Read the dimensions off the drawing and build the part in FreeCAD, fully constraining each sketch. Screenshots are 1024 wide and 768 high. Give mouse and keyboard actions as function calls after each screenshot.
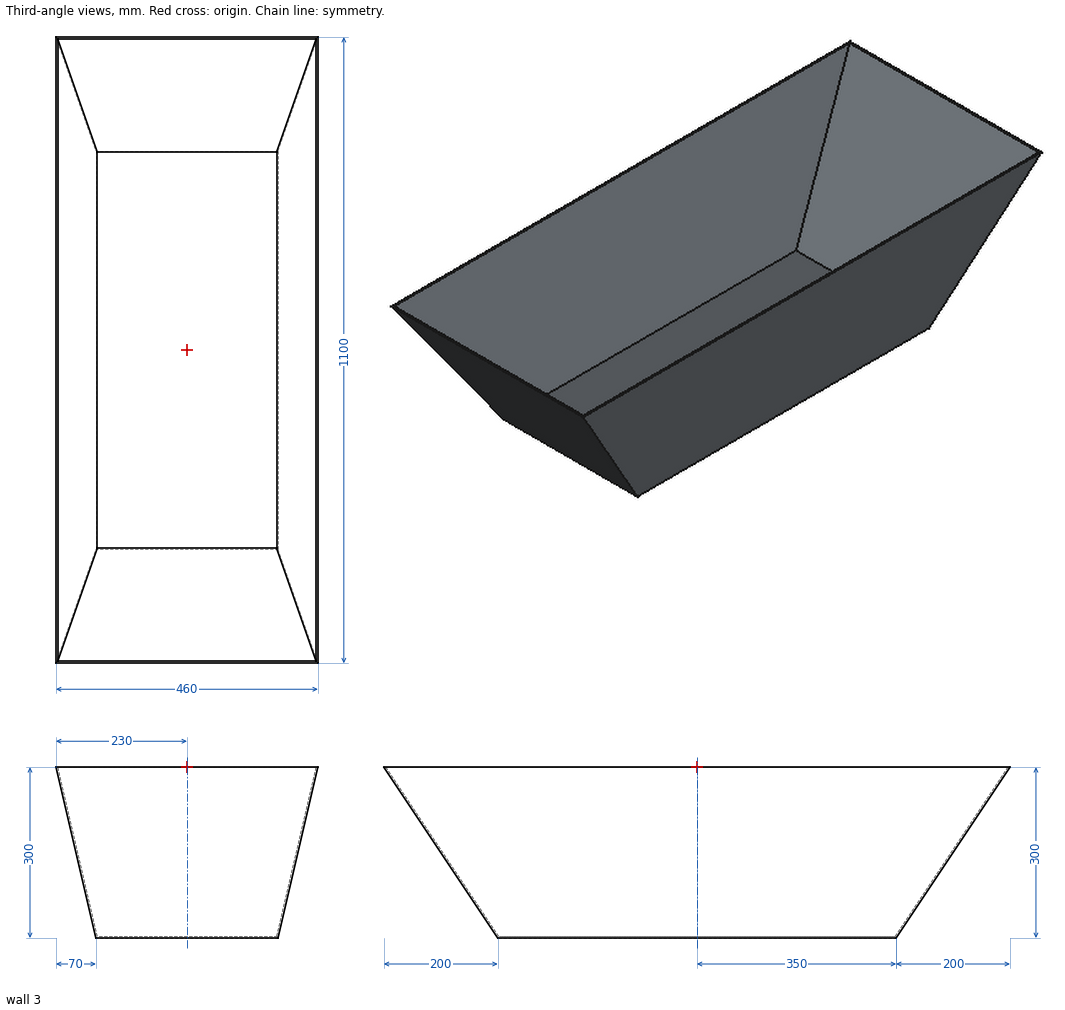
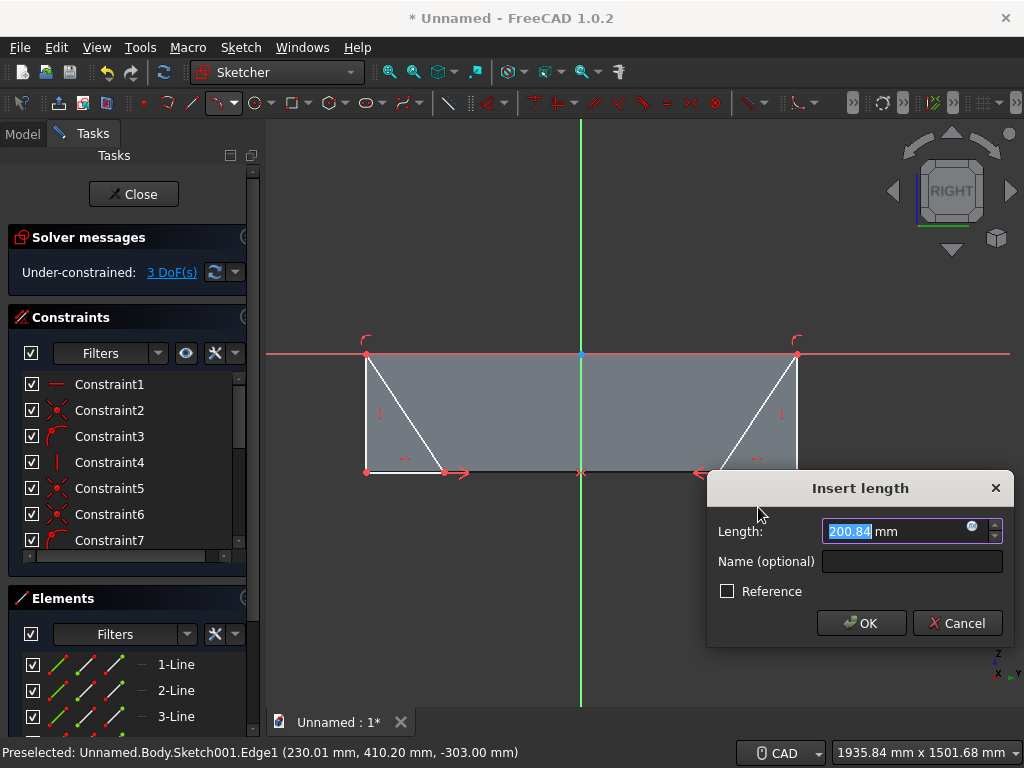
text(200)
key(Return)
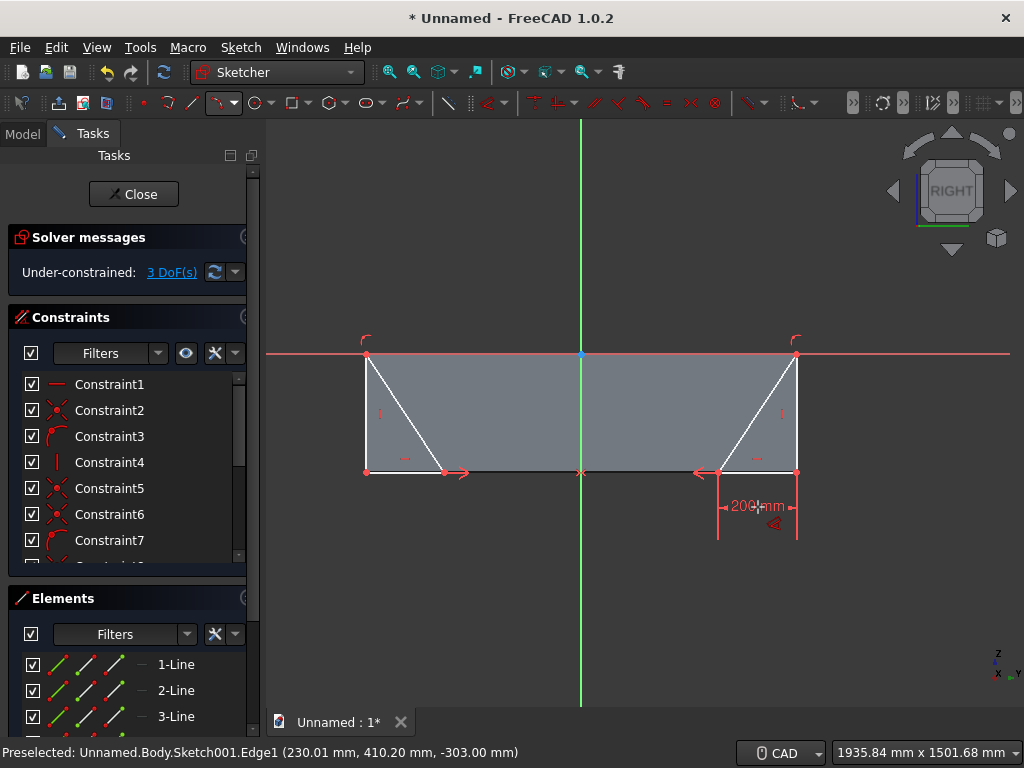
click(797, 437)
click(831, 414)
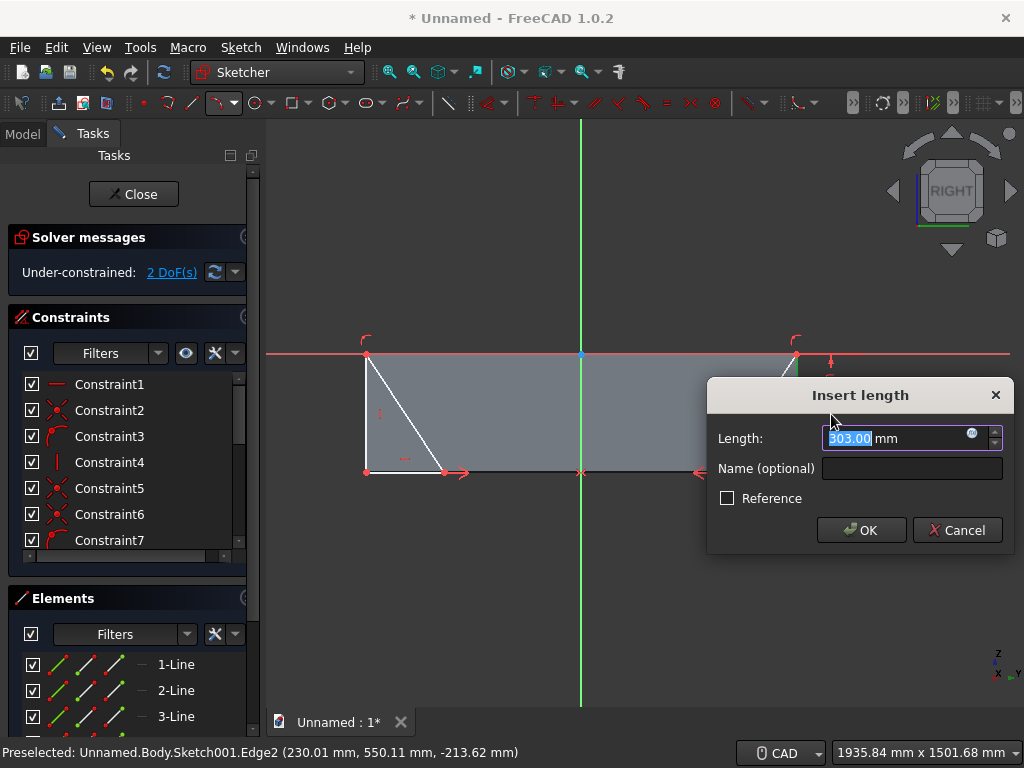
text(300)
key(Return)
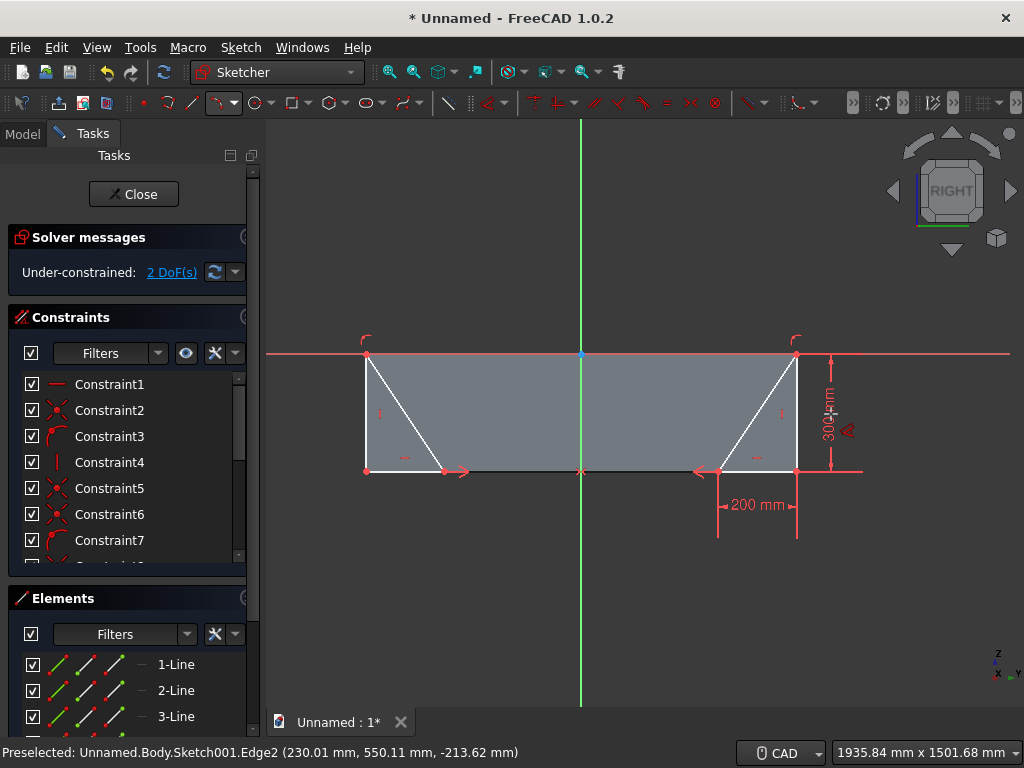
click(389, 472)
click(405, 506)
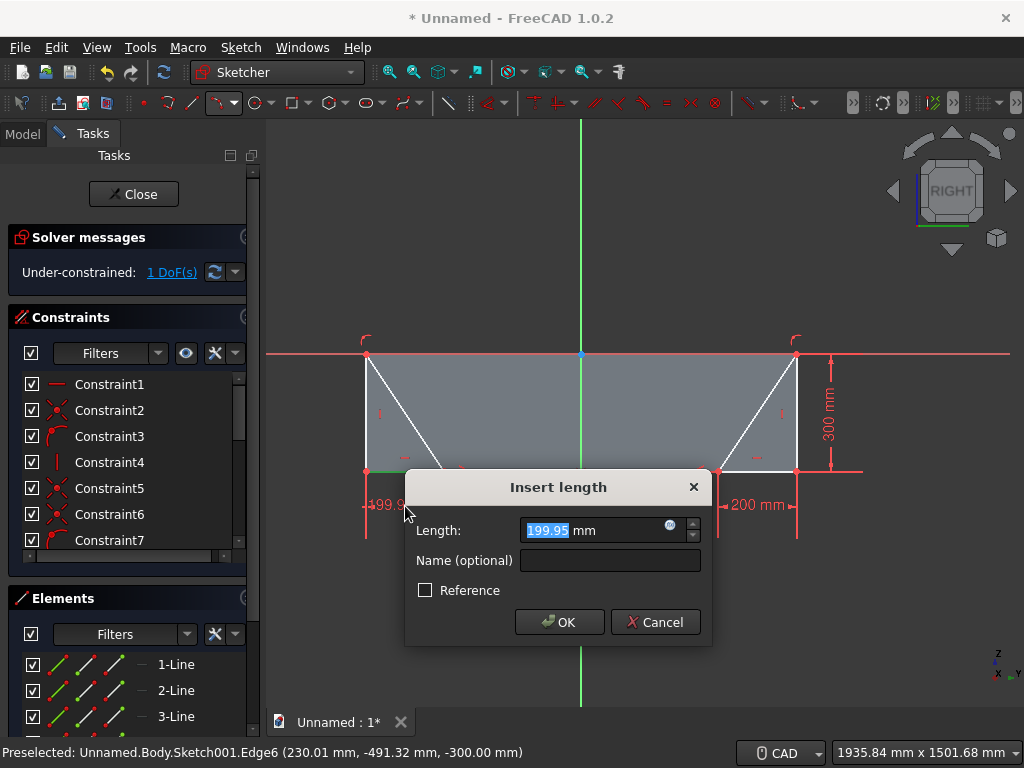
text(200)
key(Return)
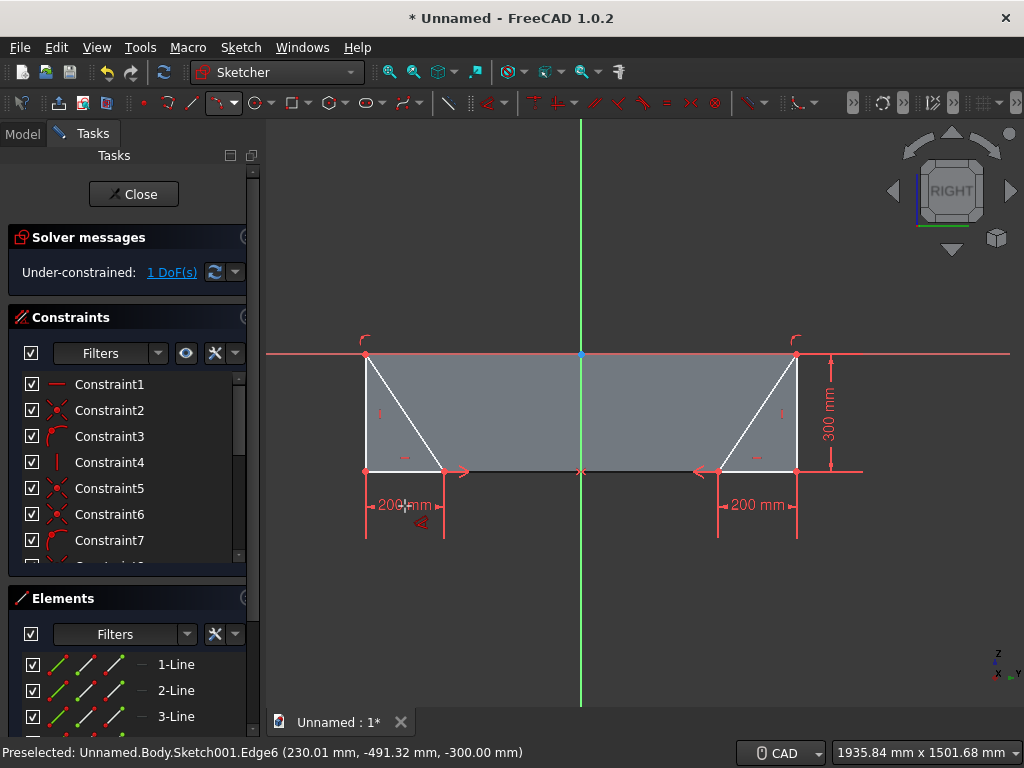
click(718, 472)
click(650, 506)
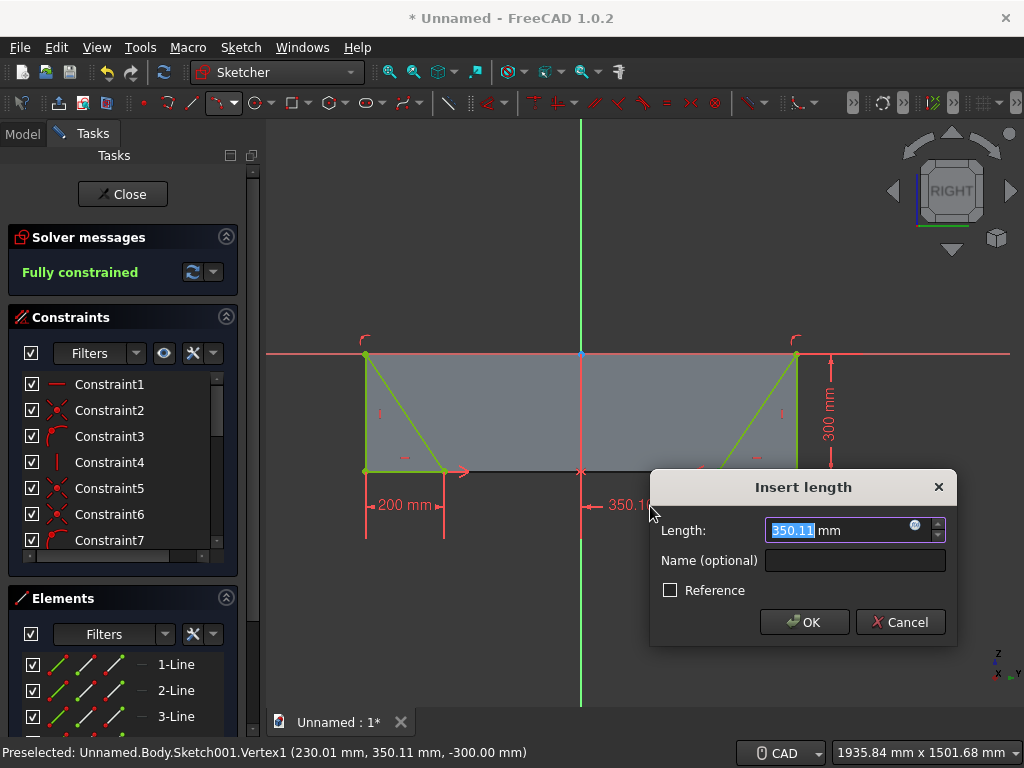
text(350)
key(Return)
key(Escape)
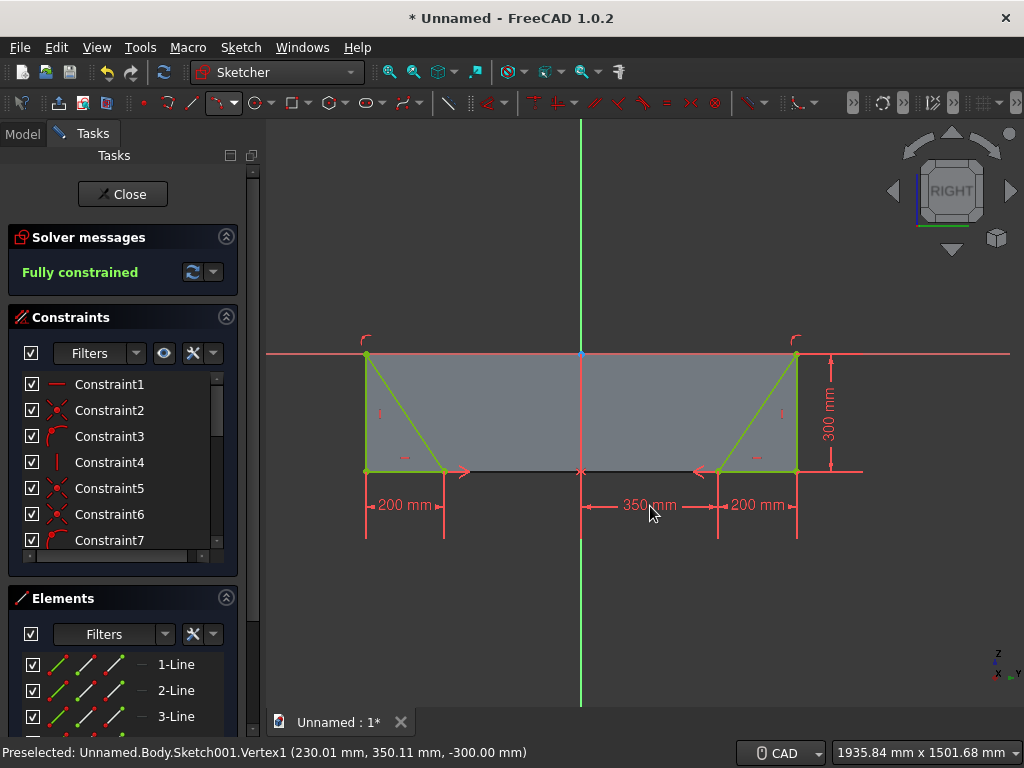
click(123, 194)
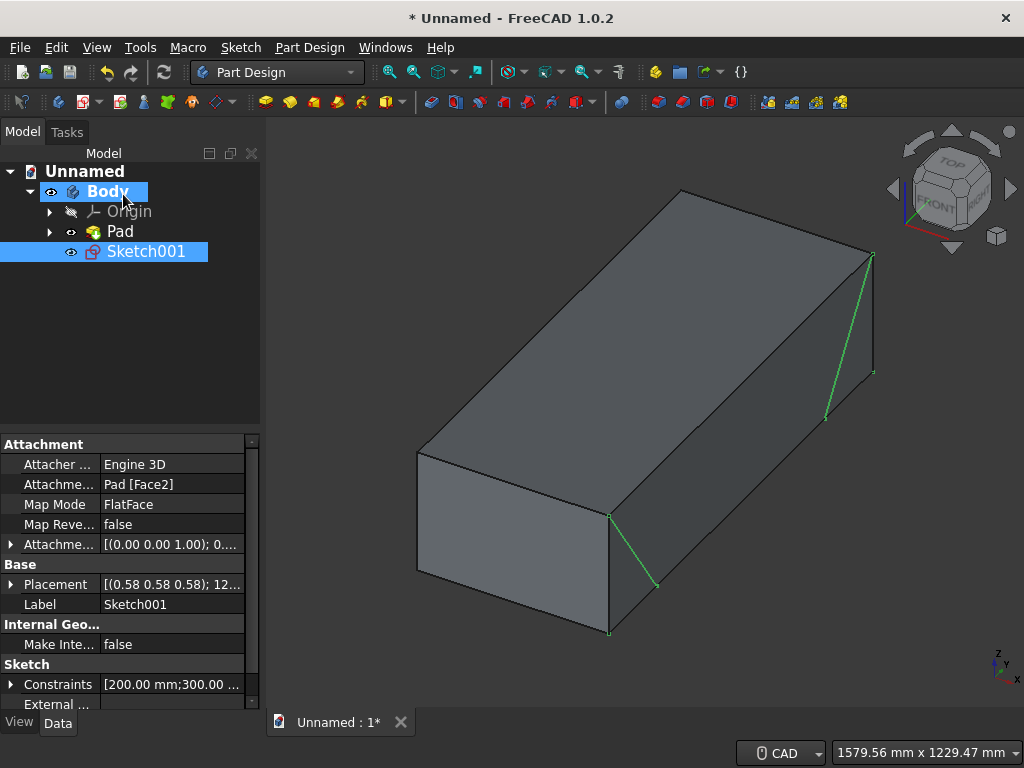
click(432, 102)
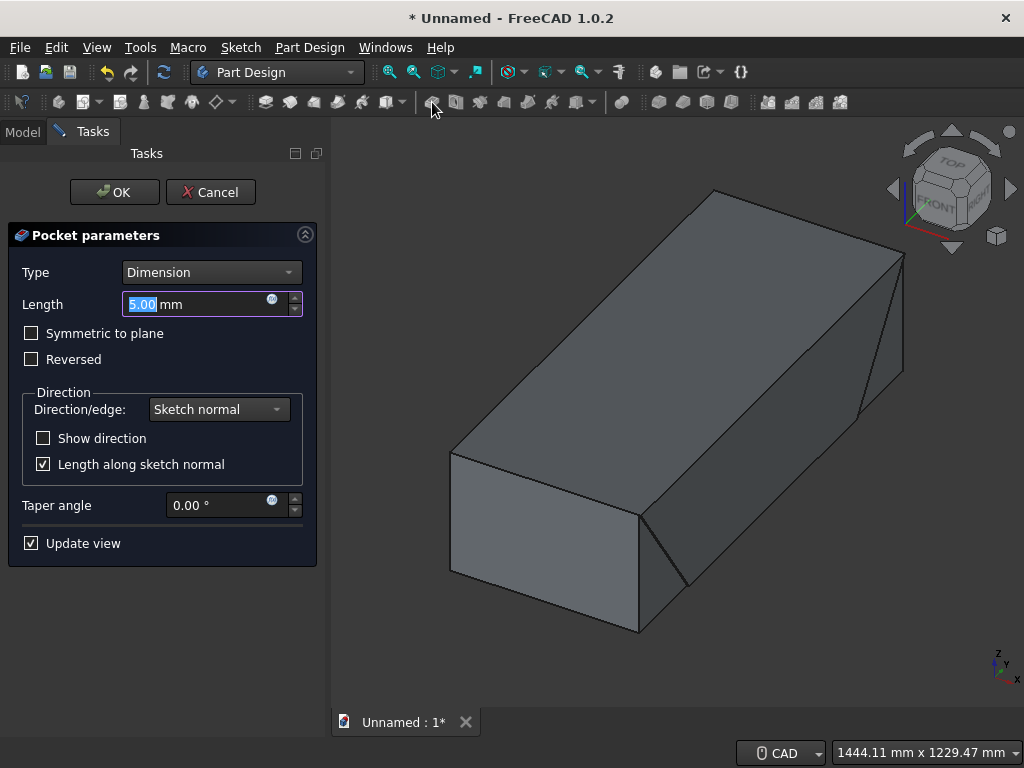
click(212, 272)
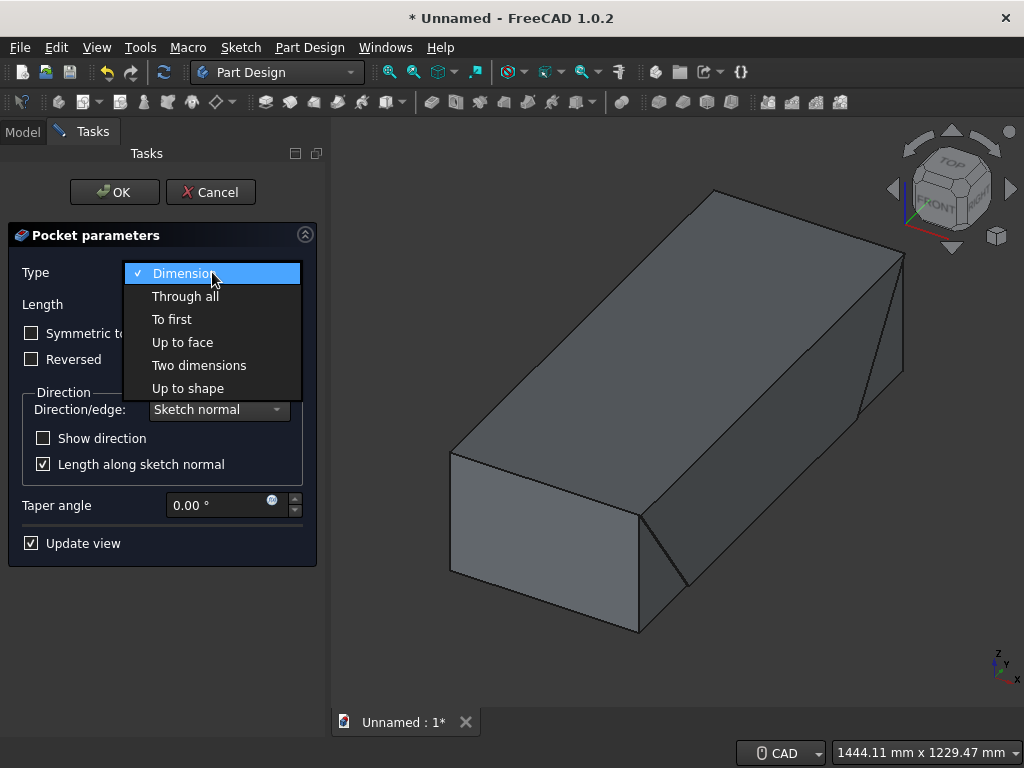
click(212, 296)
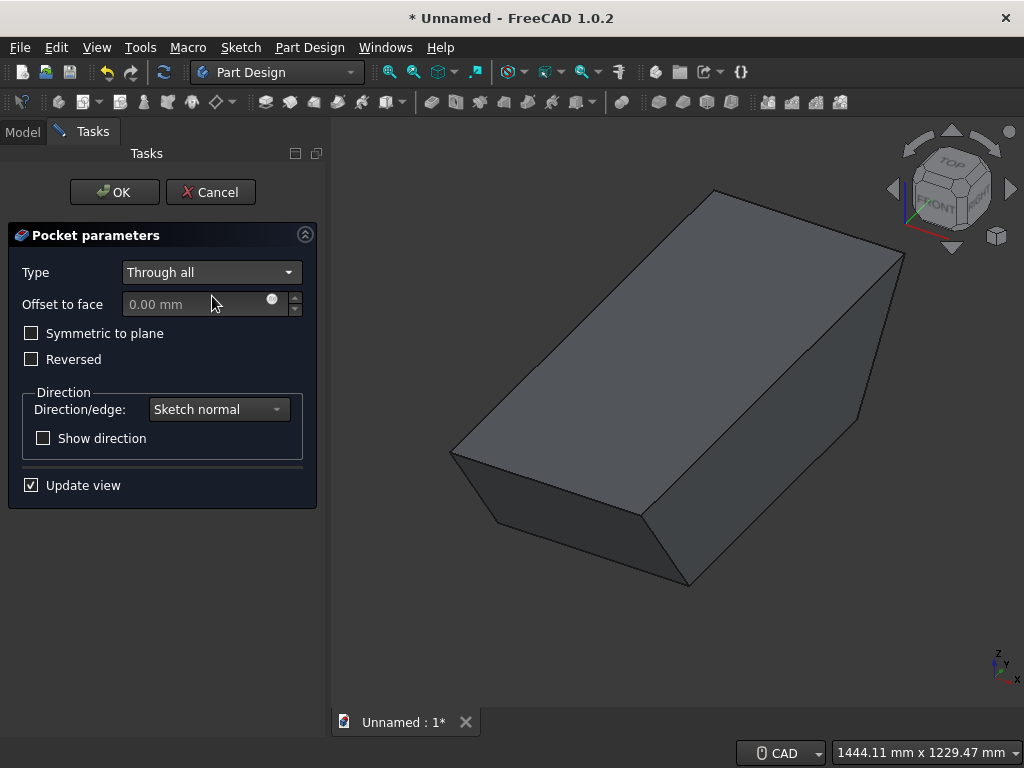
click(115, 192)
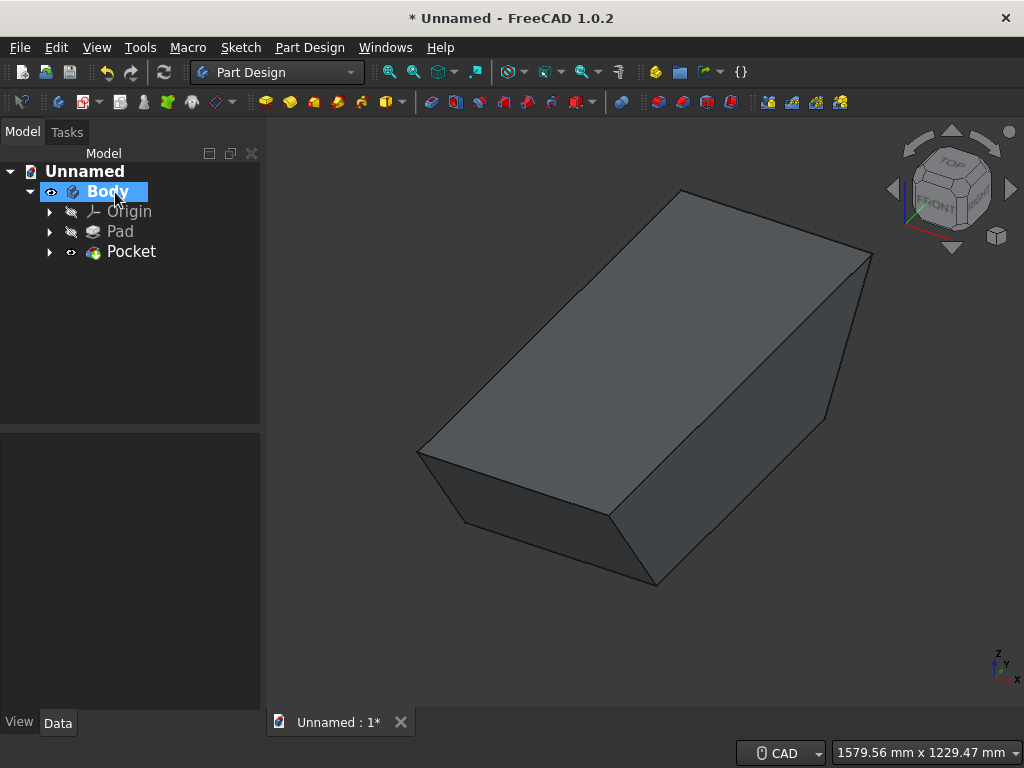
click(84, 102)